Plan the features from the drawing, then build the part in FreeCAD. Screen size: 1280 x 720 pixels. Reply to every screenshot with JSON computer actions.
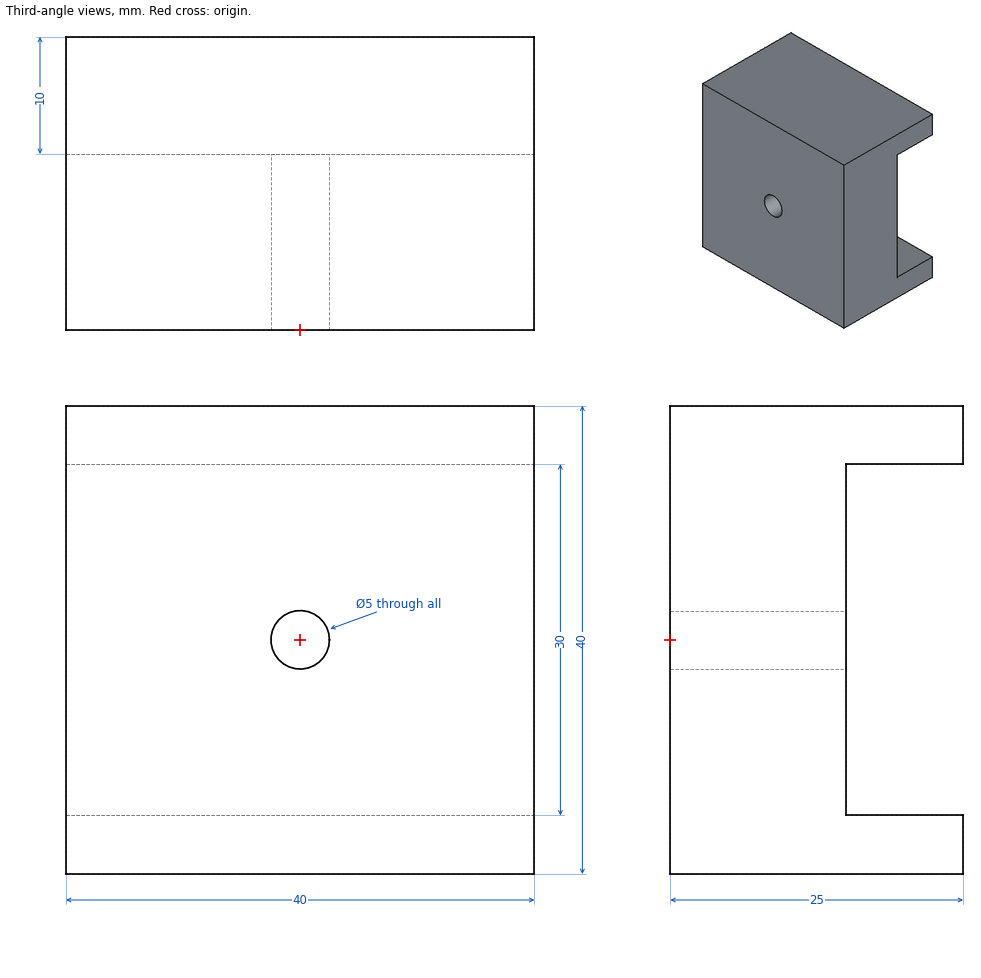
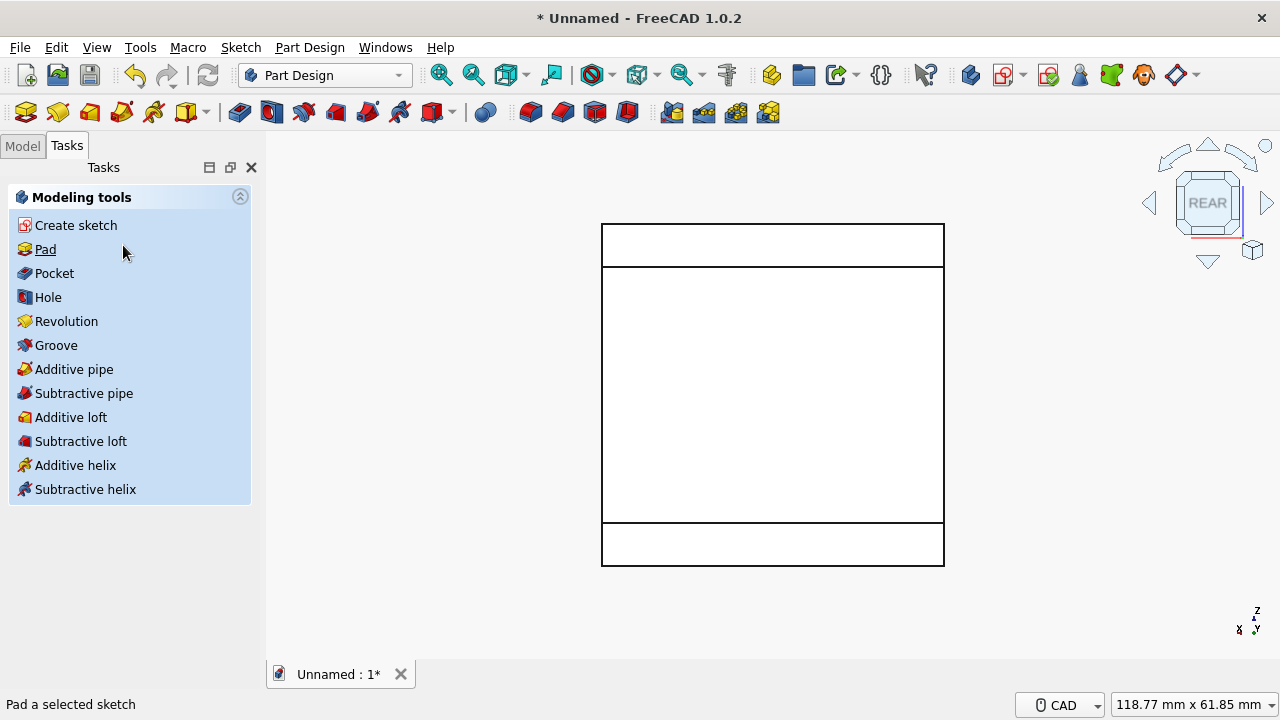
{"action": "left_click", "coordinate": [272, 112]}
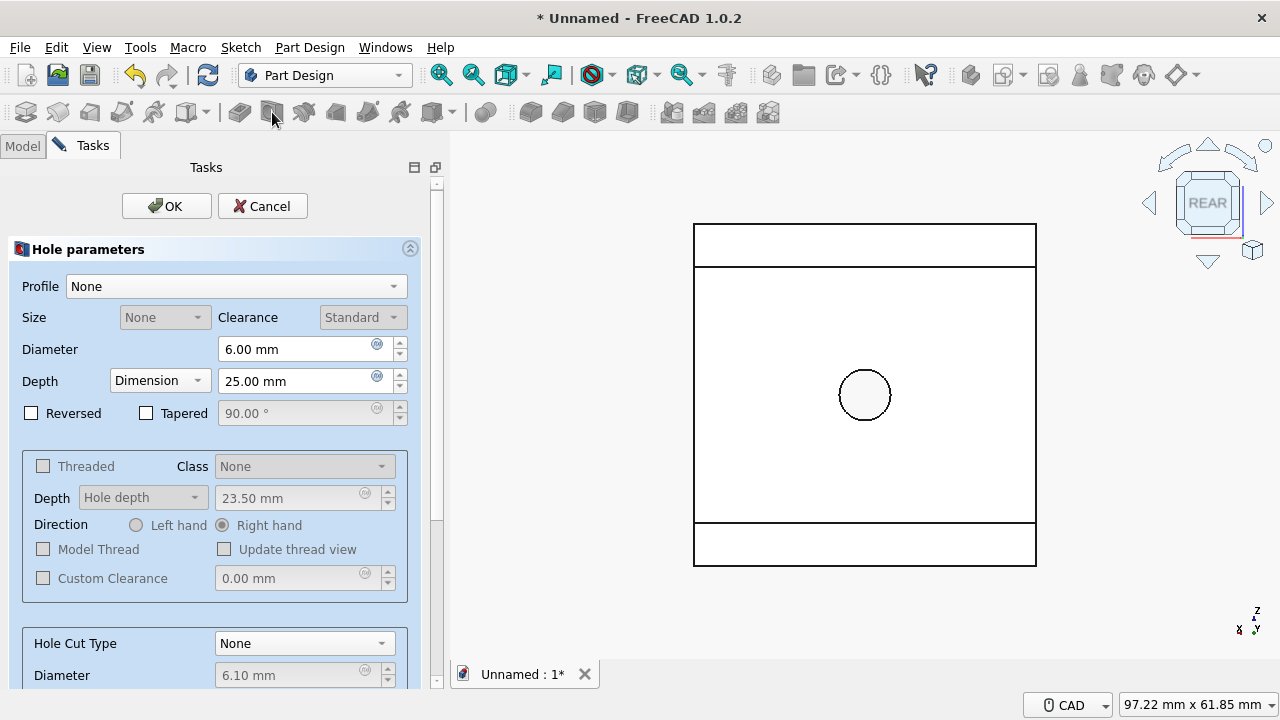
{"action": "triple_click", "coordinate": [305, 349]}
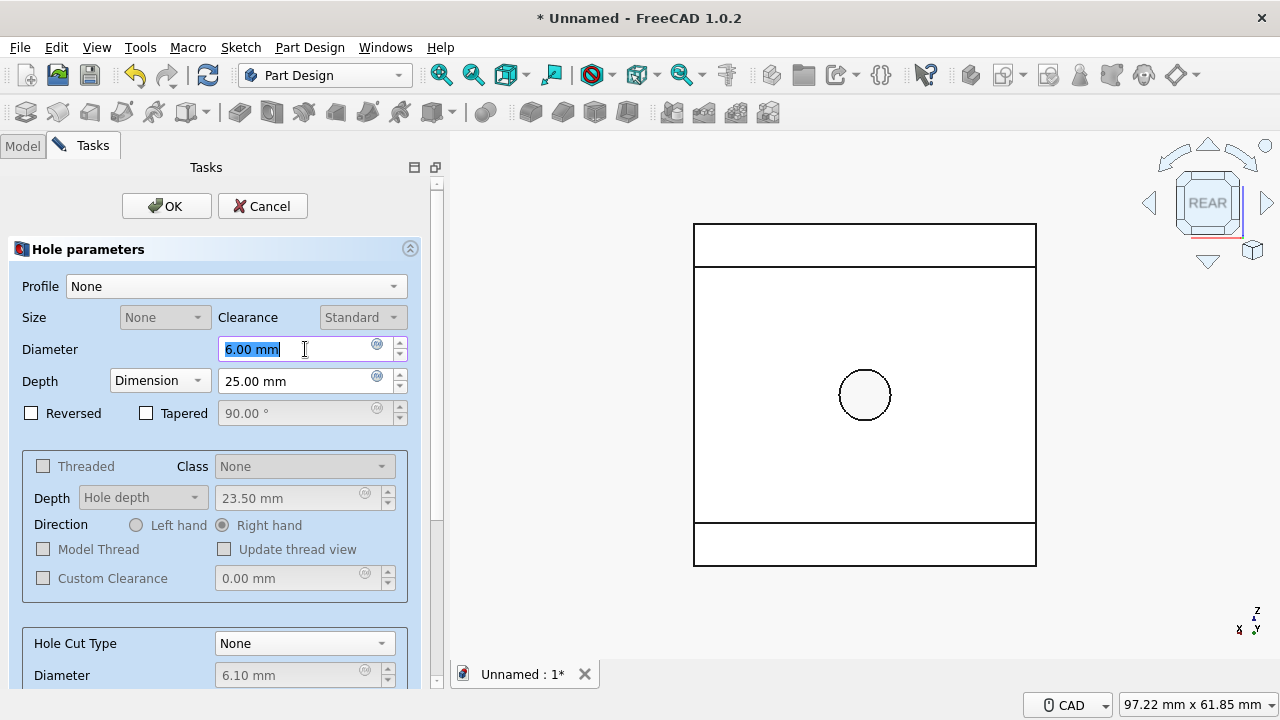
{"action": "type", "text": "5"}
{"action": "key", "text": "Tab"}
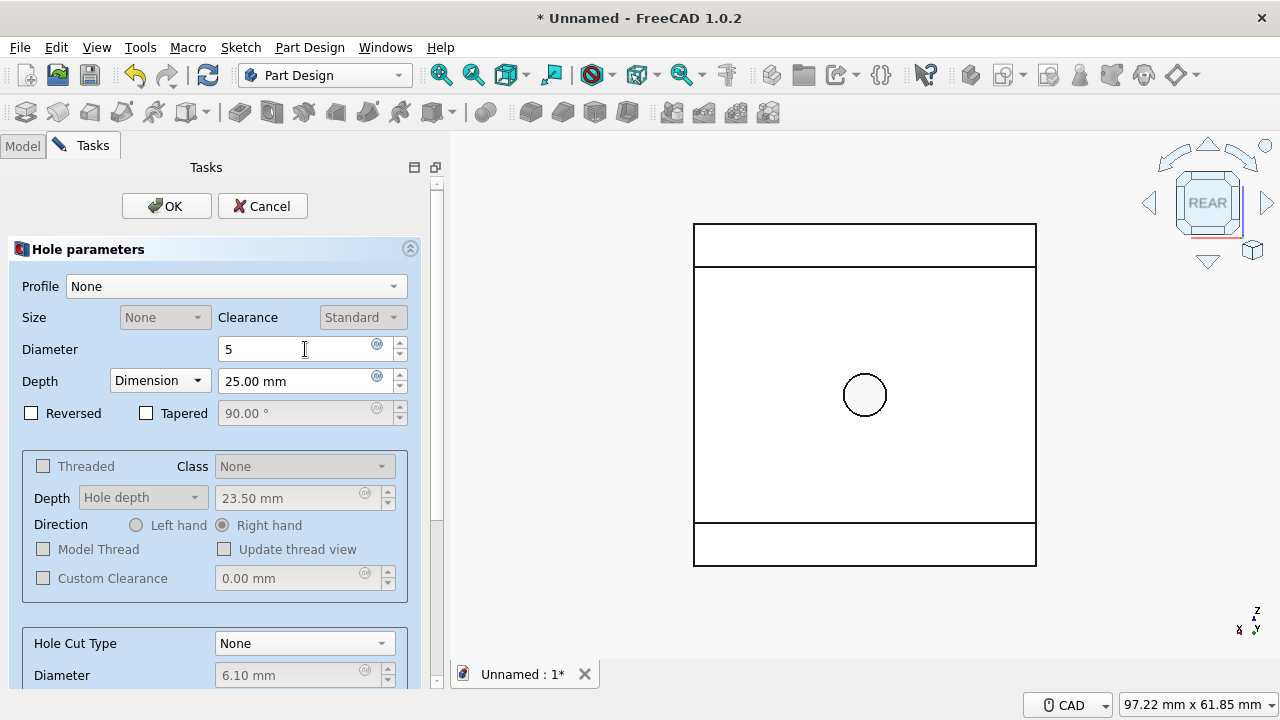
{"action": "left_click", "coordinate": [161, 380]}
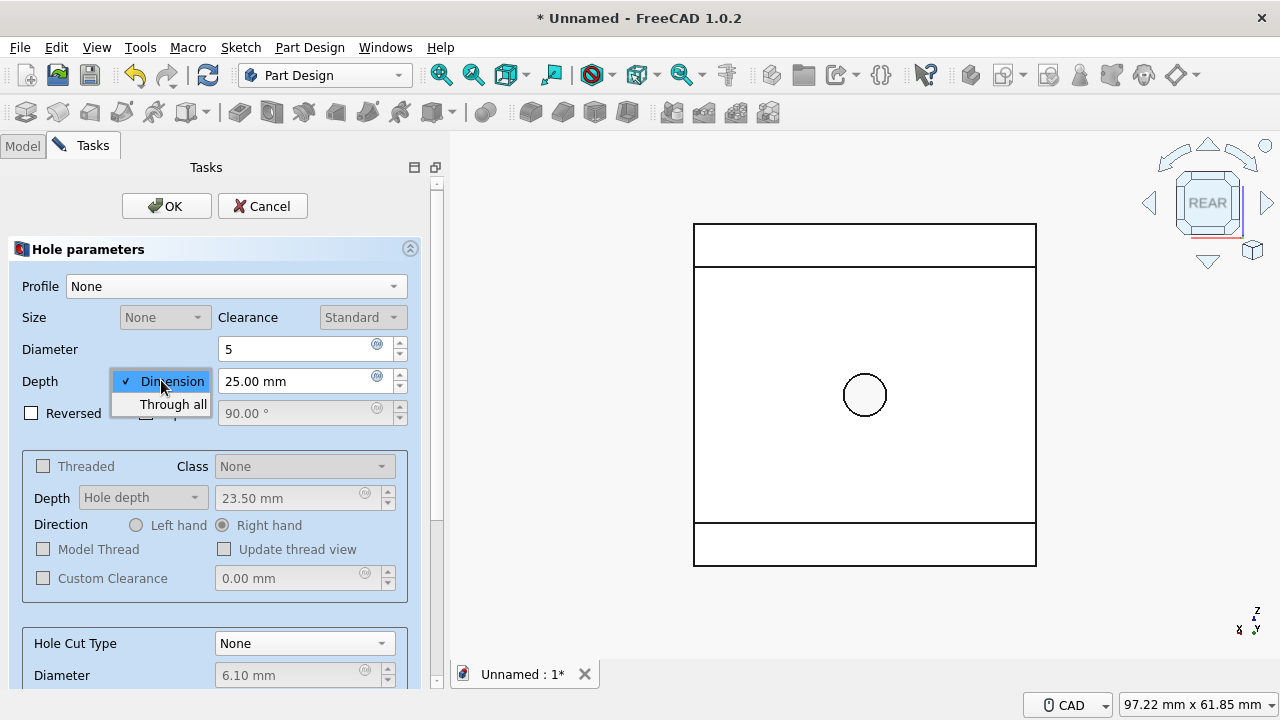
{"action": "left_click", "coordinate": [160, 404]}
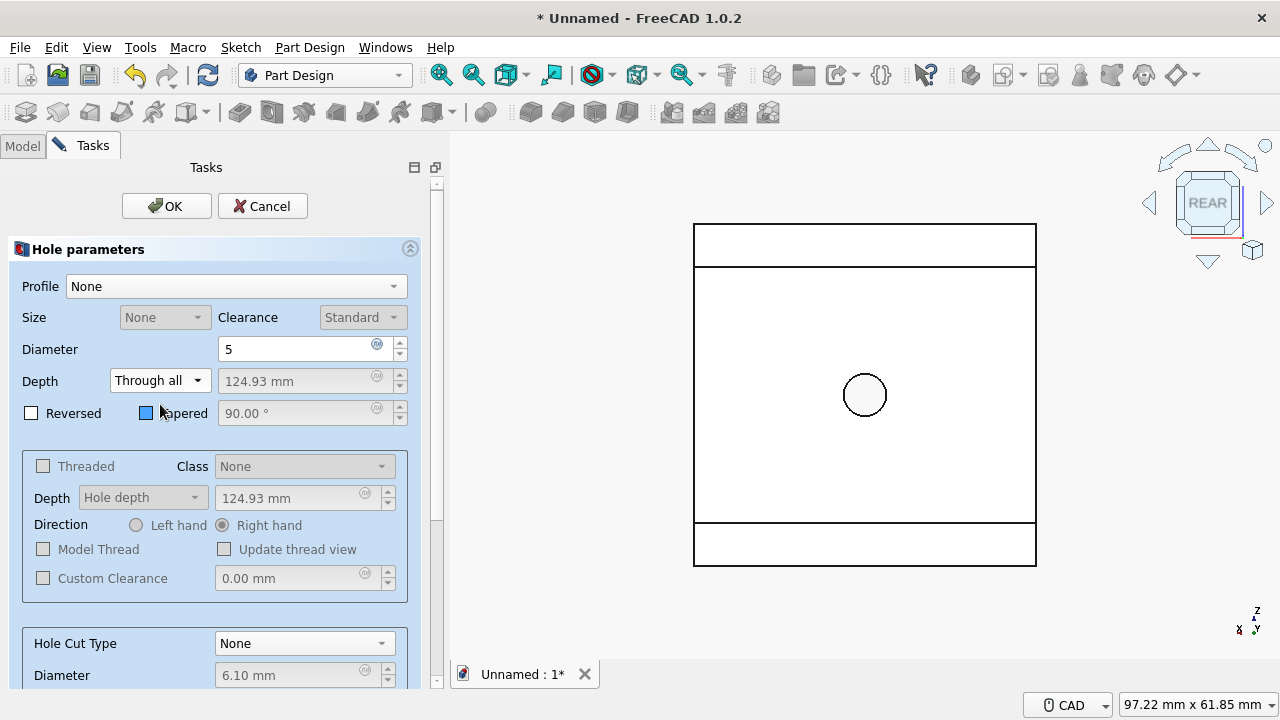
{"action": "left_click", "coordinate": [167, 206]}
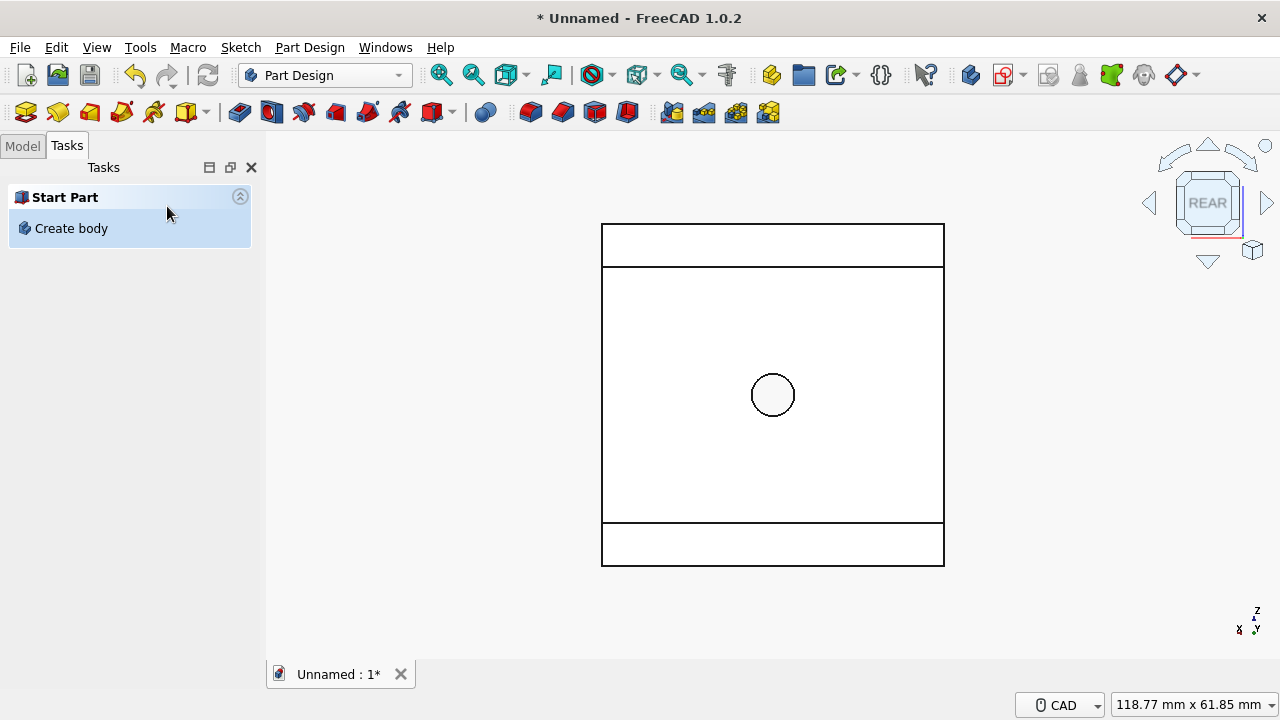
{"action": "key", "text": "0"}